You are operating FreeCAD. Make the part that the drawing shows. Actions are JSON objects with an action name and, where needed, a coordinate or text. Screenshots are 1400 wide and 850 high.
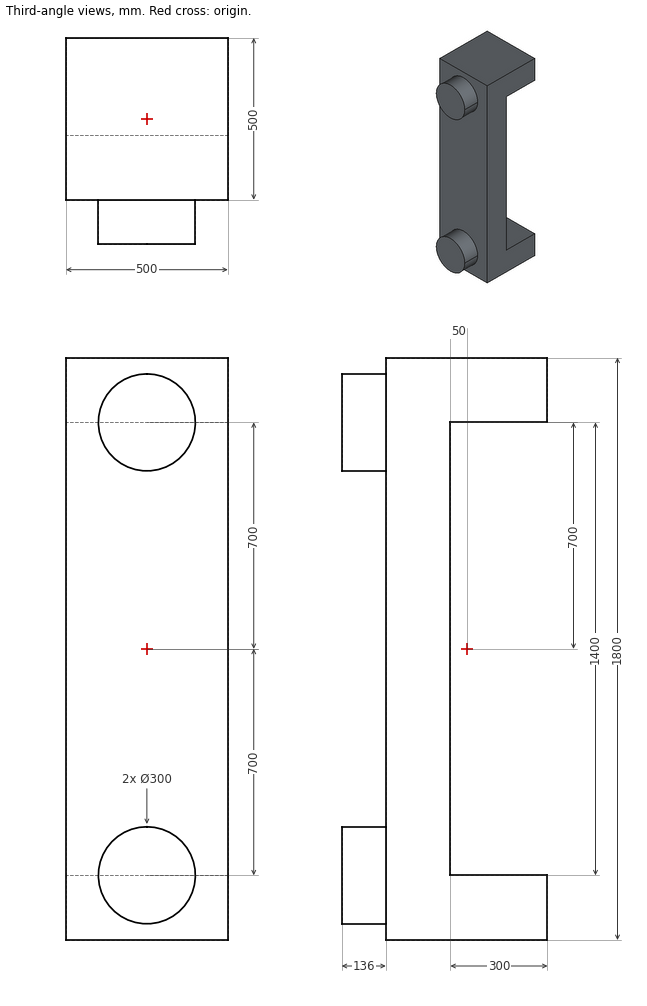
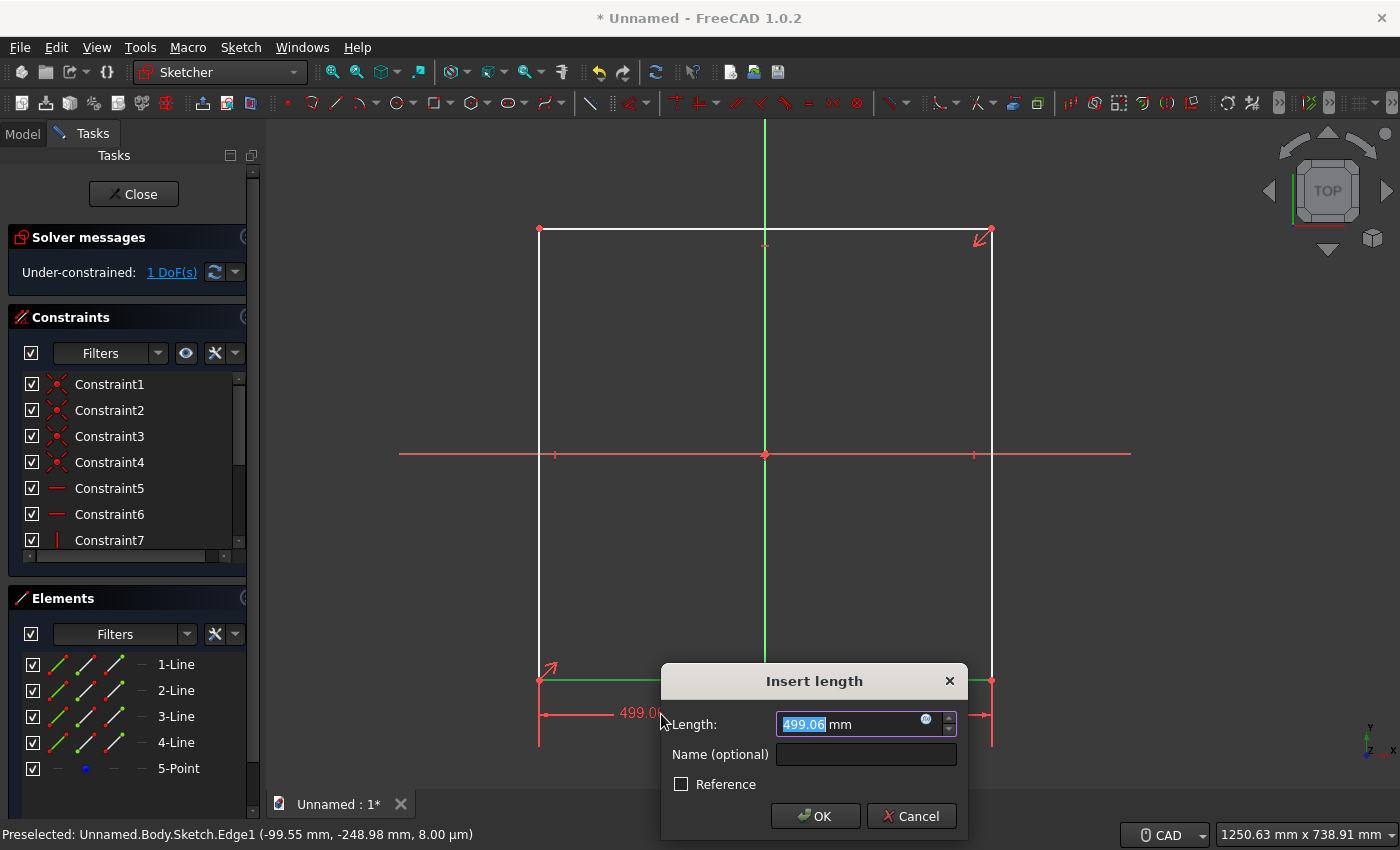
{"action": "type", "text": "500"}
{"action": "key", "text": "Return"}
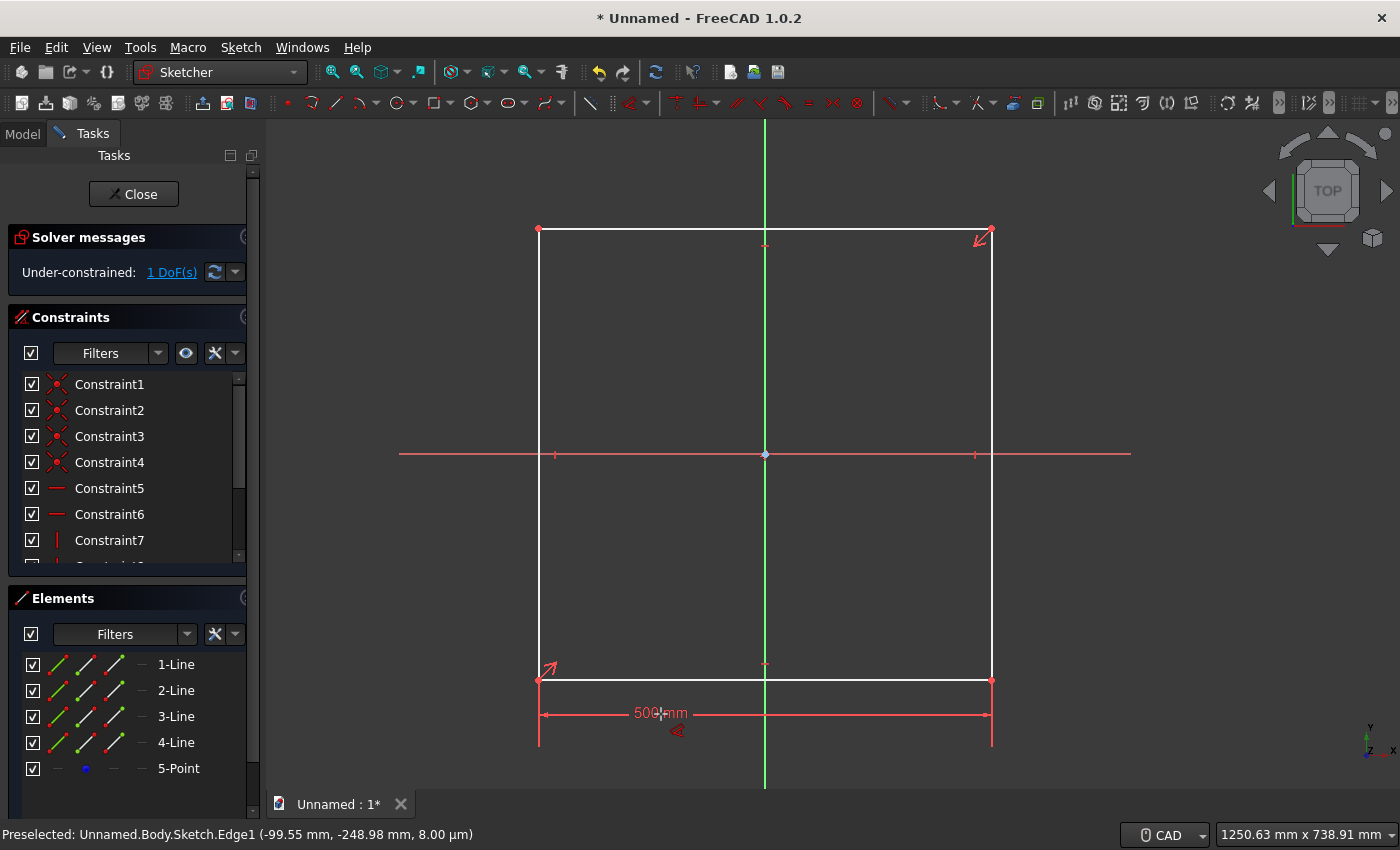
{"action": "left_click", "coordinate": [992, 545]}
{"action": "left_click", "coordinate": [1026, 351]}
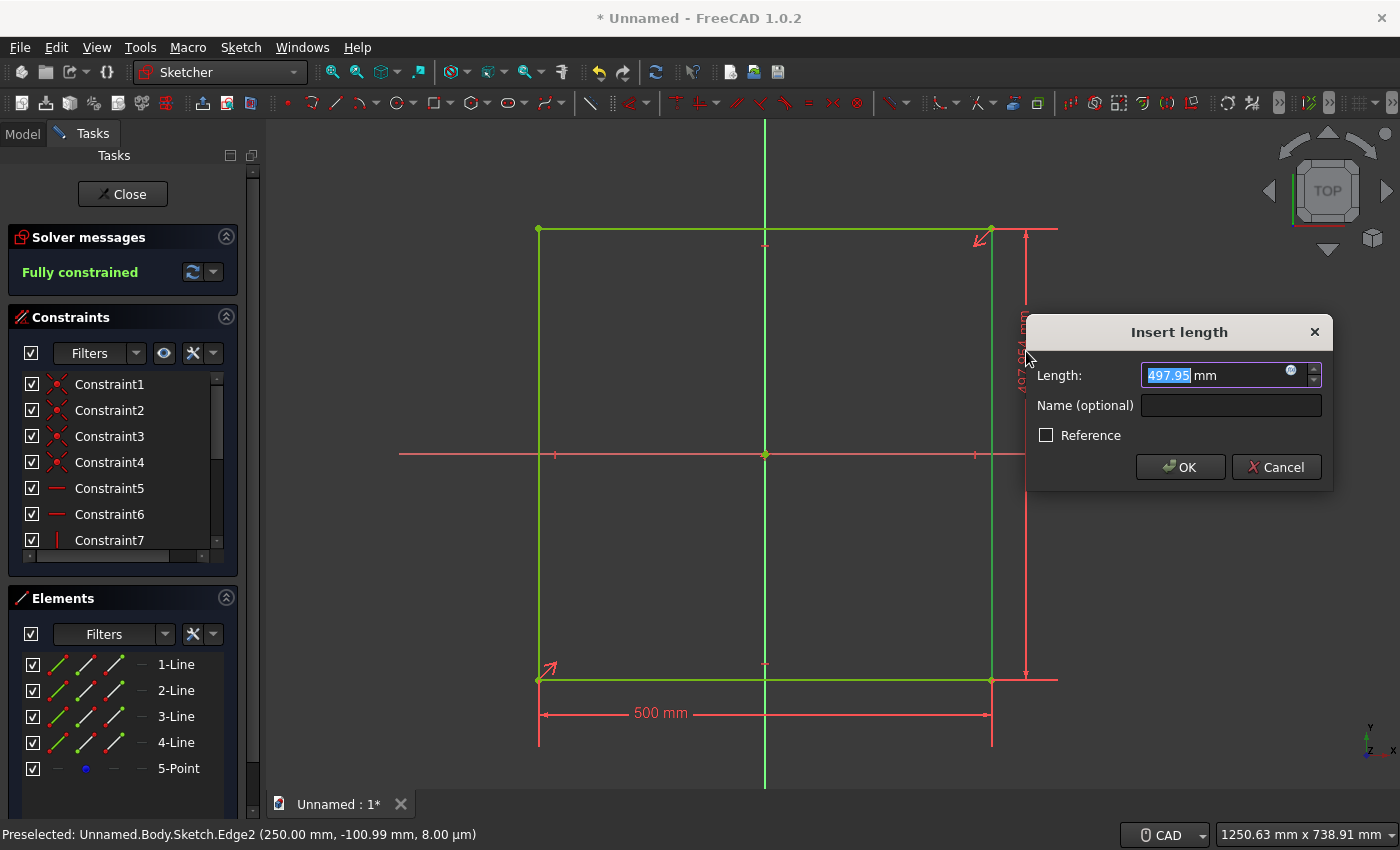
{"action": "type", "text": "500"}
{"action": "key", "text": "Return"}
{"action": "key", "text": "Escape"}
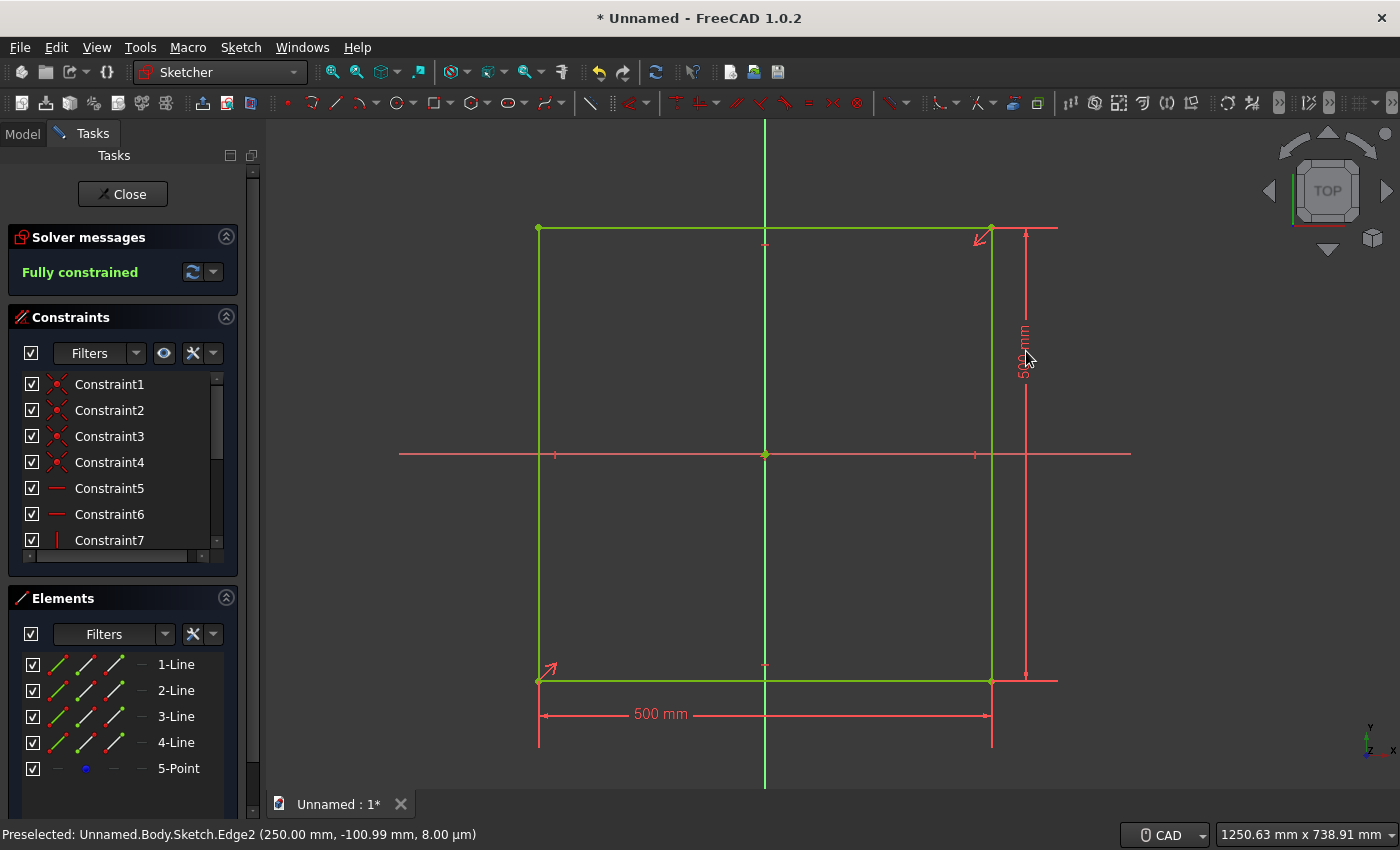
{"action": "left_click", "coordinate": [123, 194]}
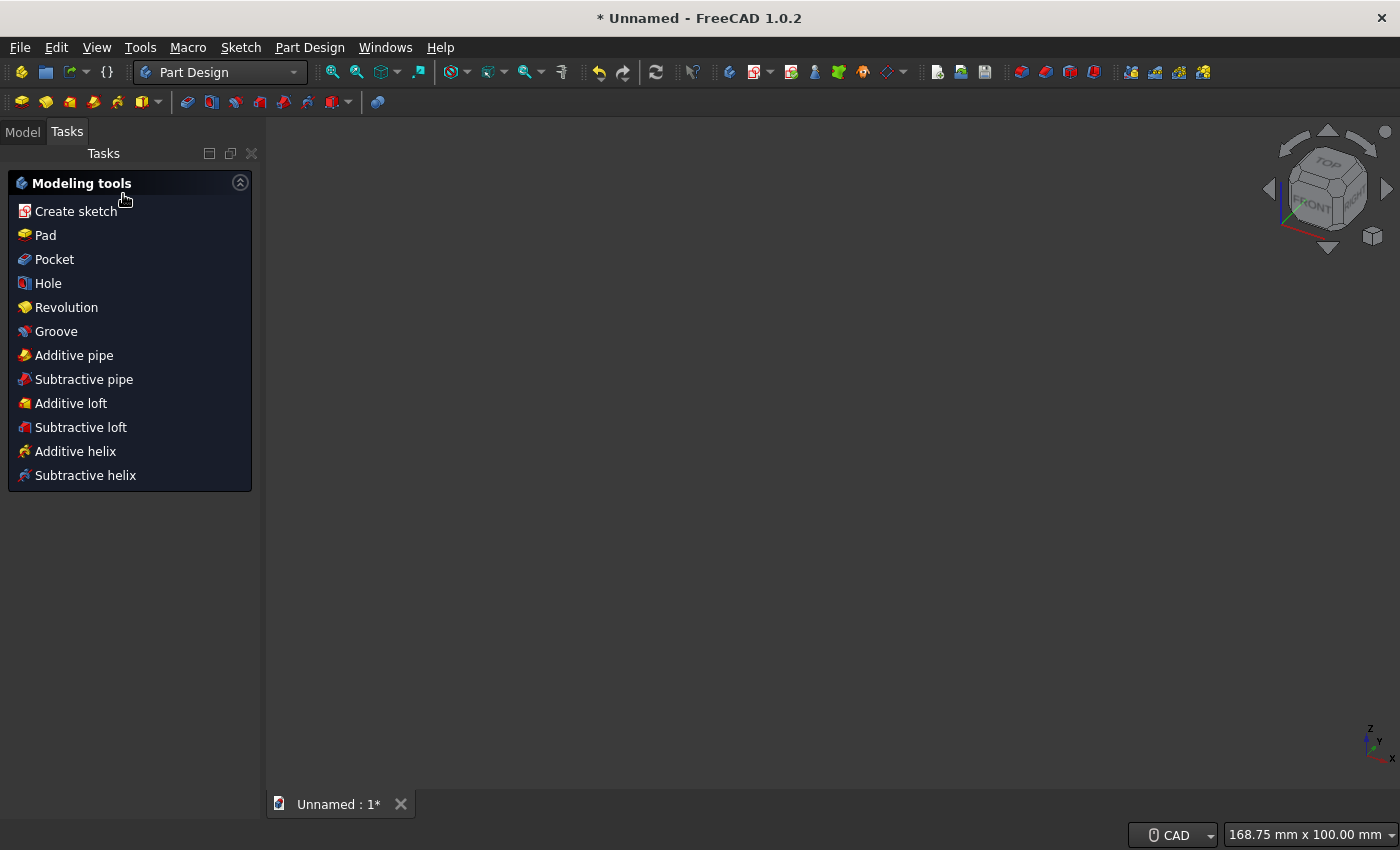
{"action": "left_click", "coordinate": [22, 102]}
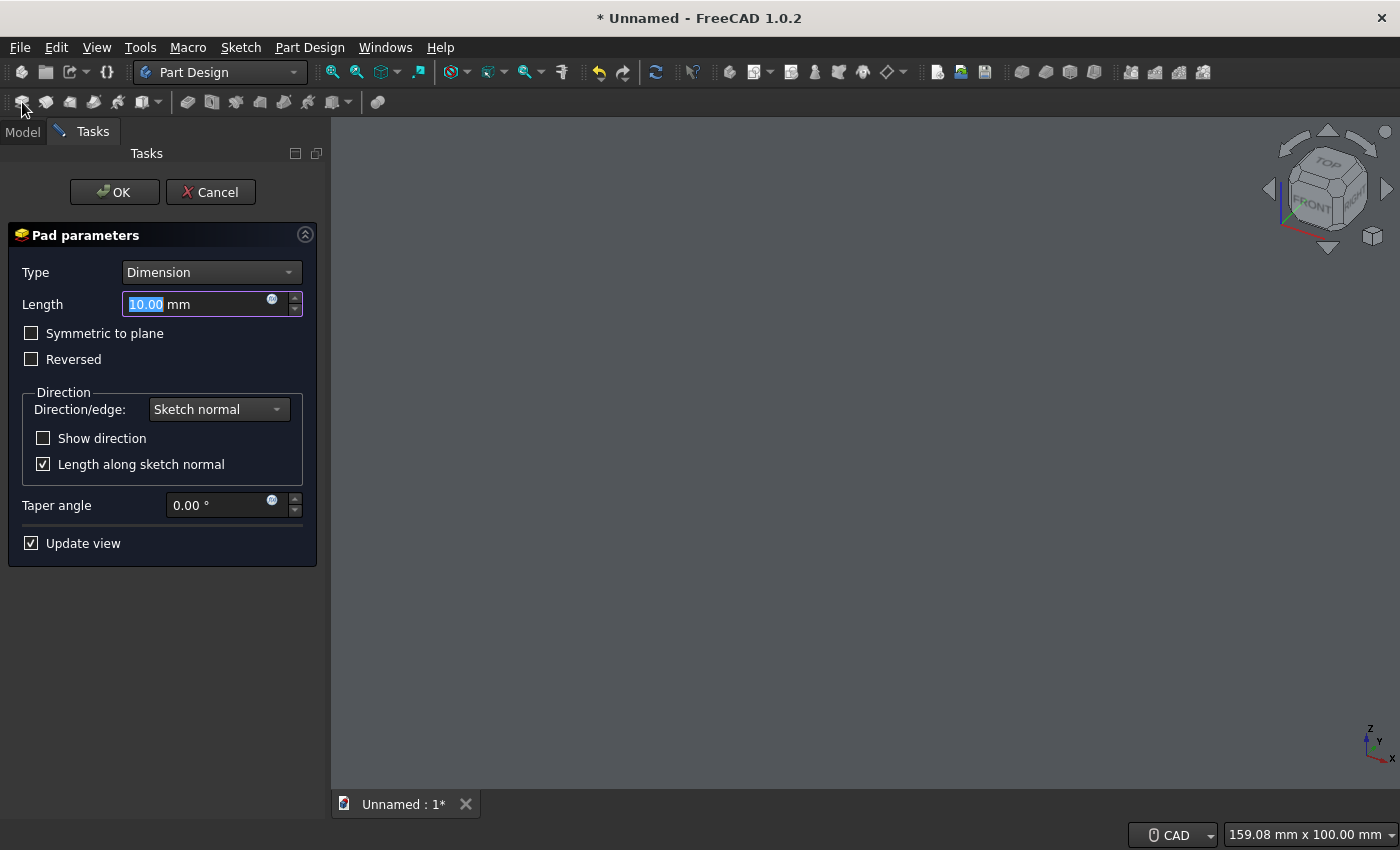
{"action": "type", "text": "1800"}
{"action": "key", "text": "Tab"}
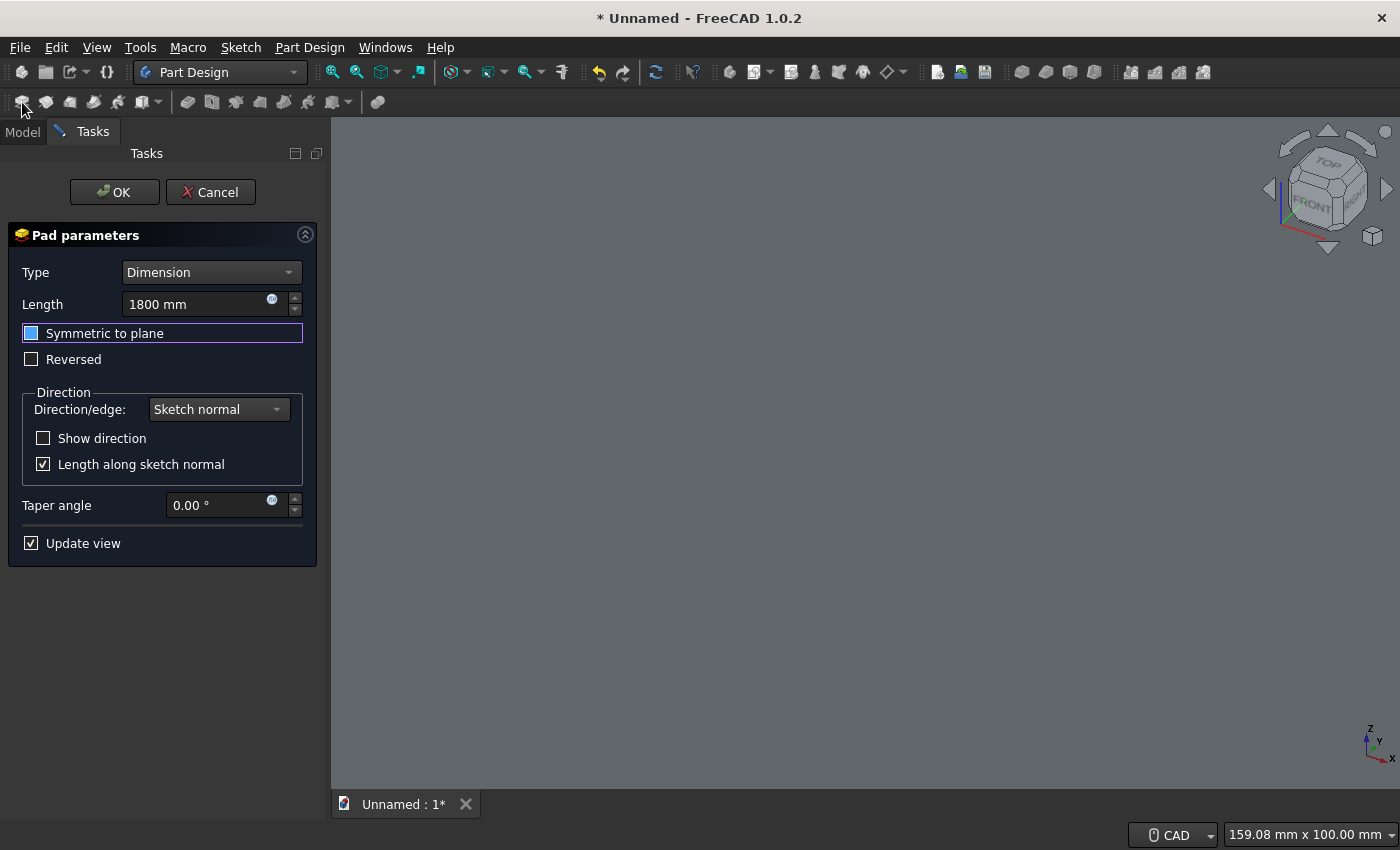
{"action": "left_click", "coordinate": [30, 333]}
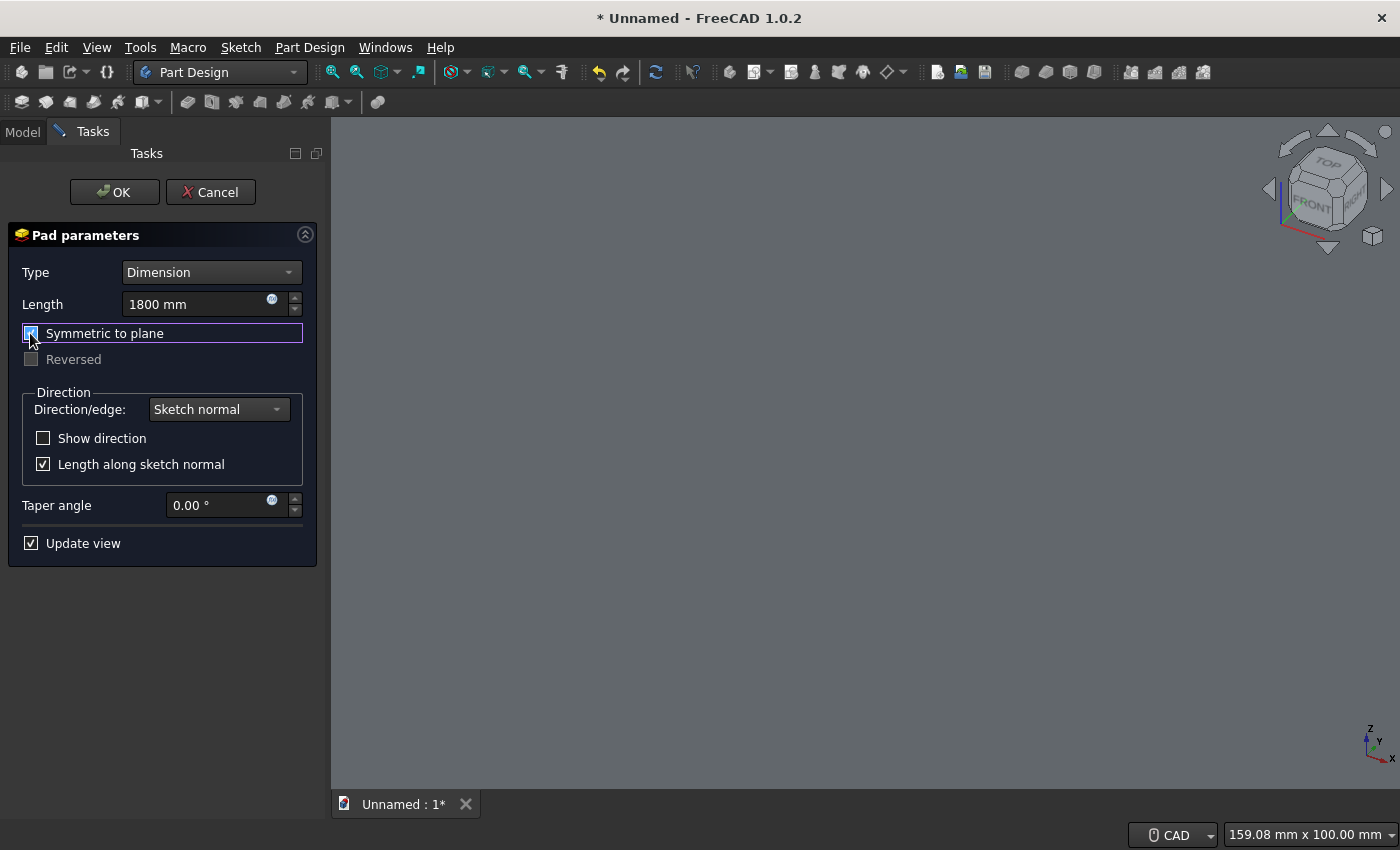
{"action": "left_click", "coordinate": [115, 192]}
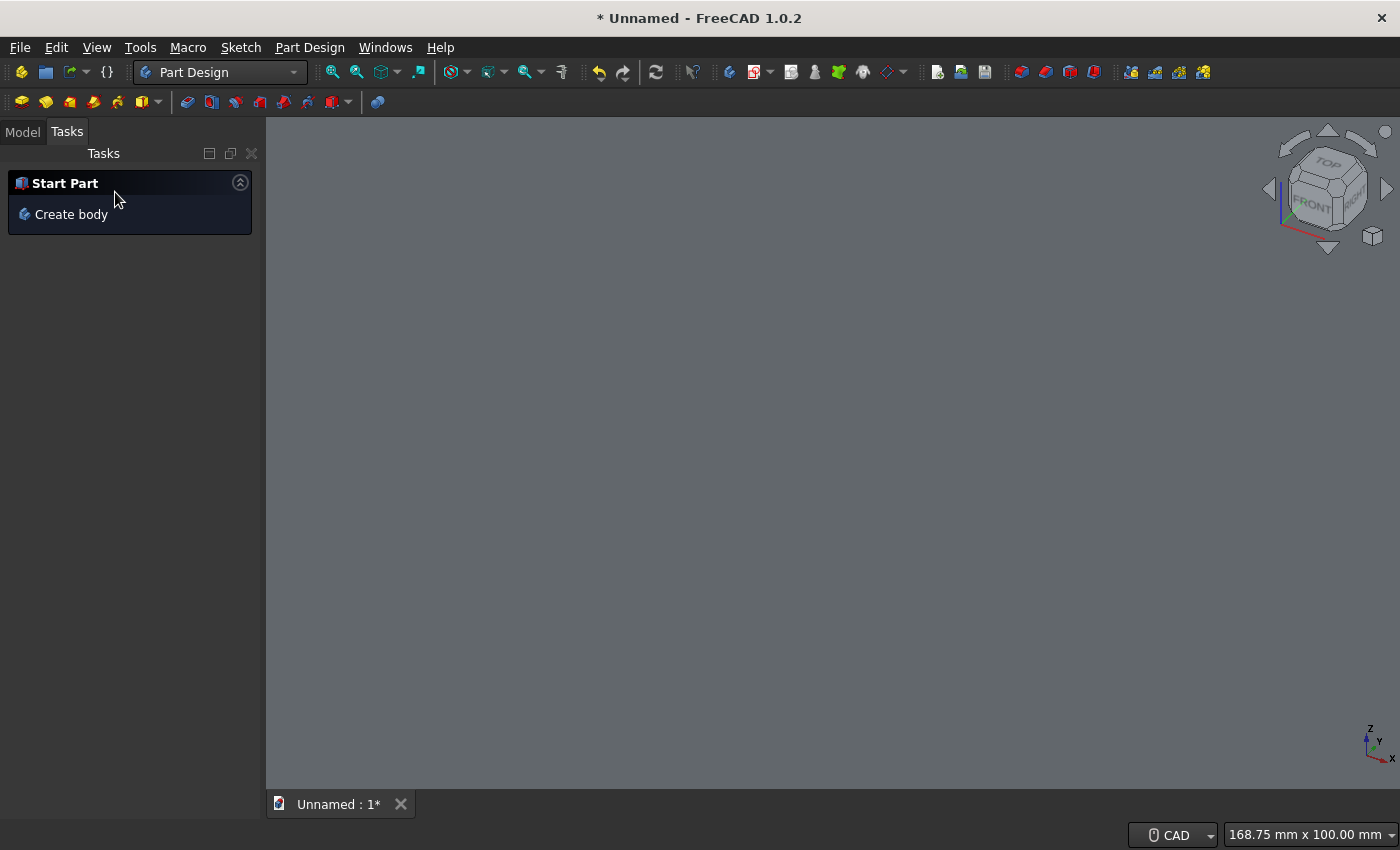
{"action": "left_click", "coordinate": [334, 72]}